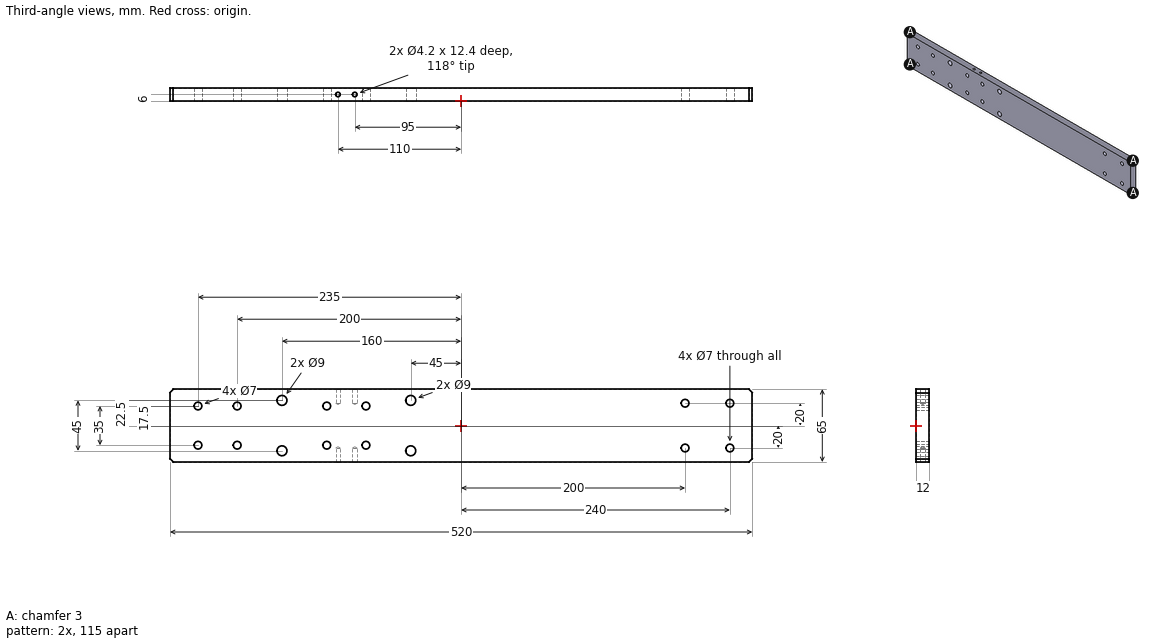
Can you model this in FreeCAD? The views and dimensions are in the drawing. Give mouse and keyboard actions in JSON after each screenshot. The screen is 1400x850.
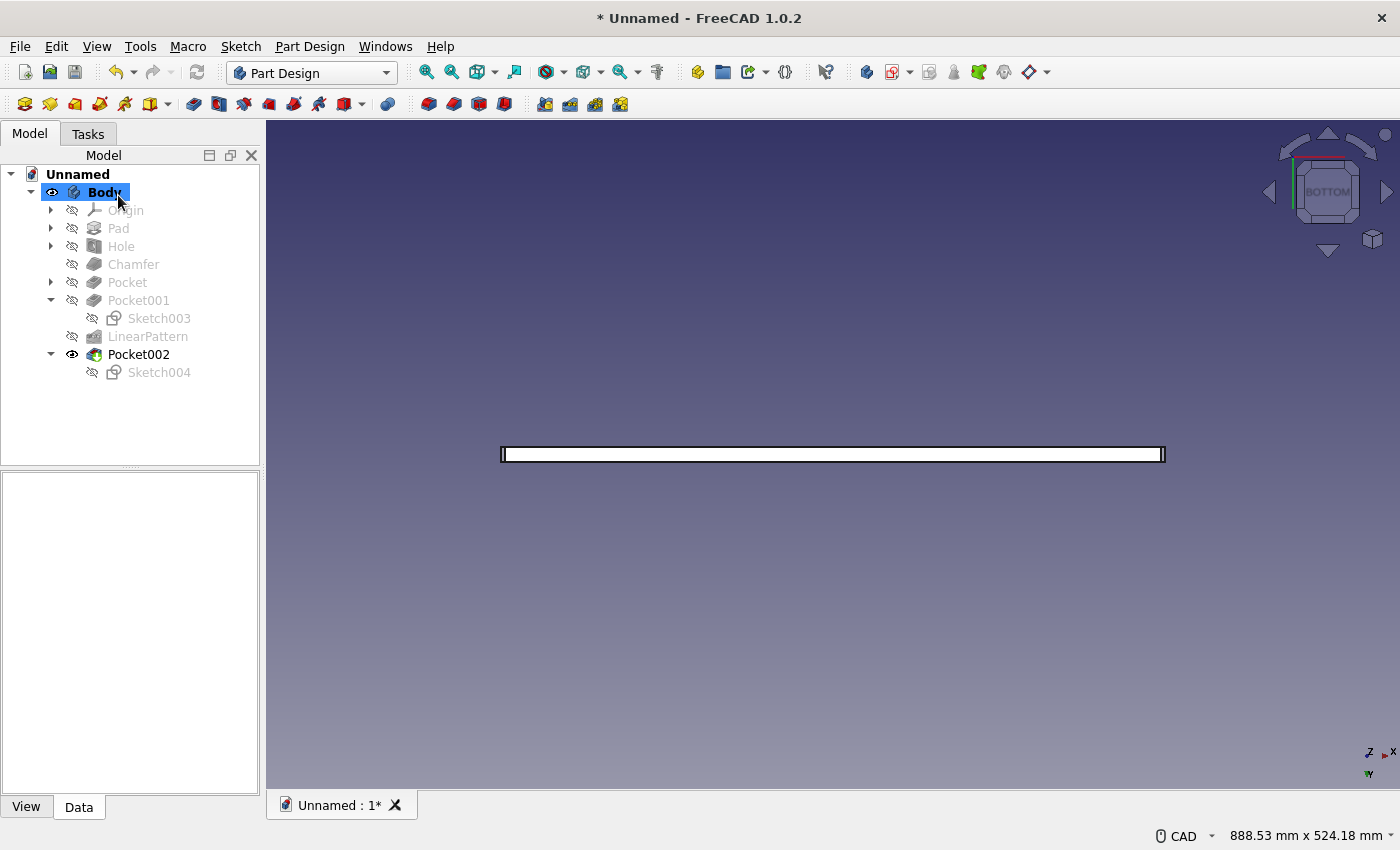
{"action": "left_click", "coordinate": [1114, 454]}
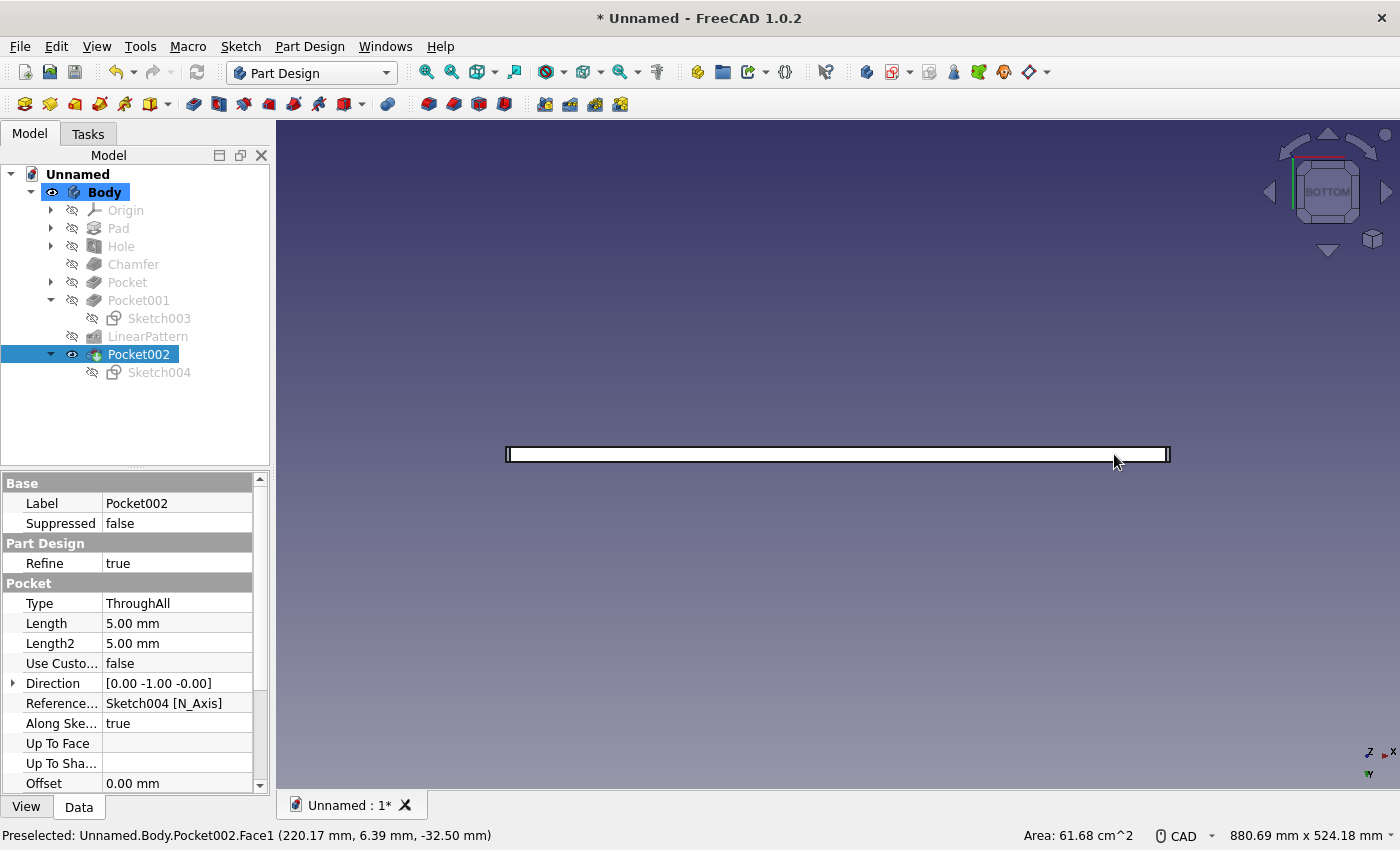
{"action": "left_click", "coordinate": [892, 72]}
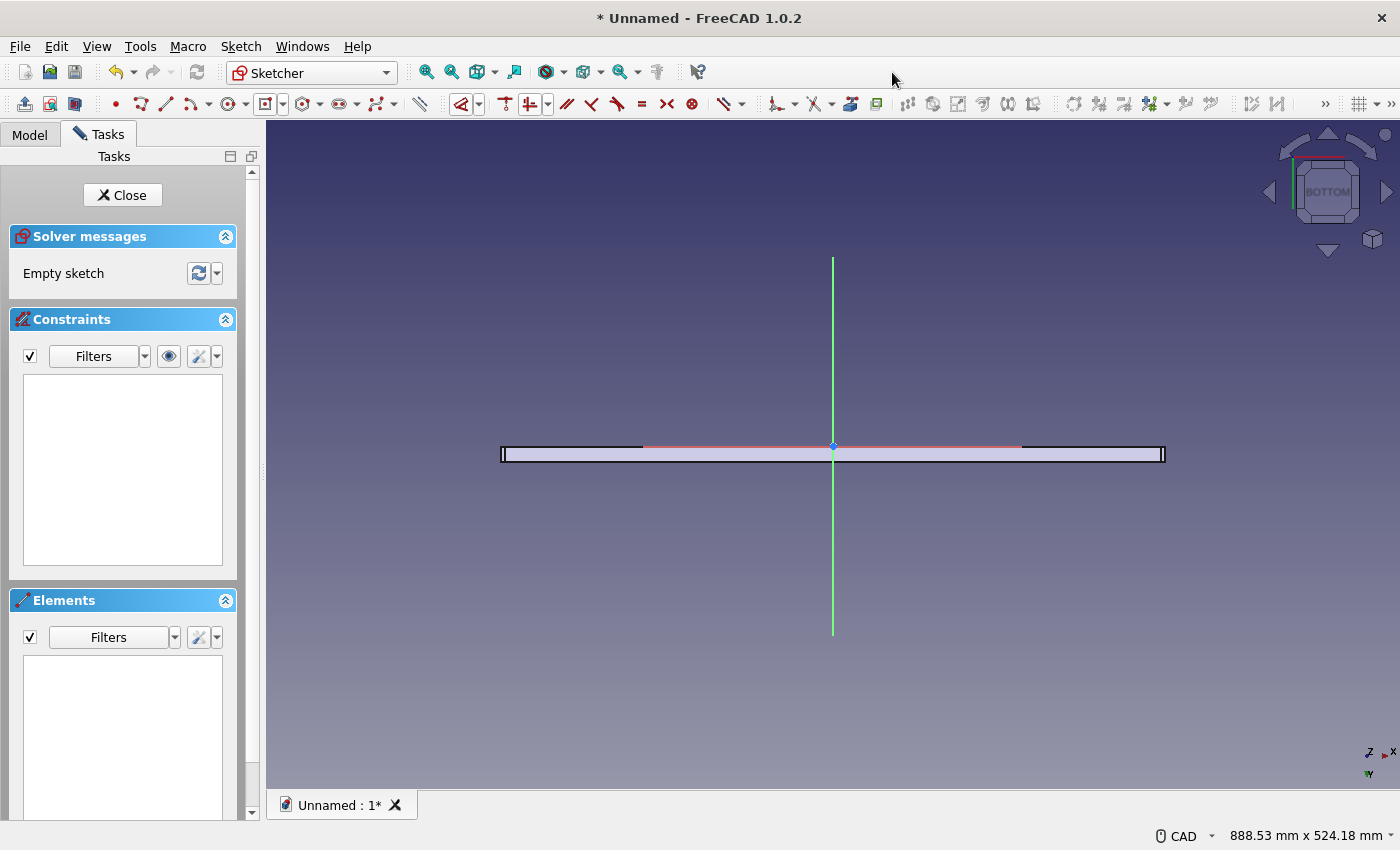
{"action": "scroll", "coordinate": [699, 455], "scroll_direction": "up", "scroll_amount": 15}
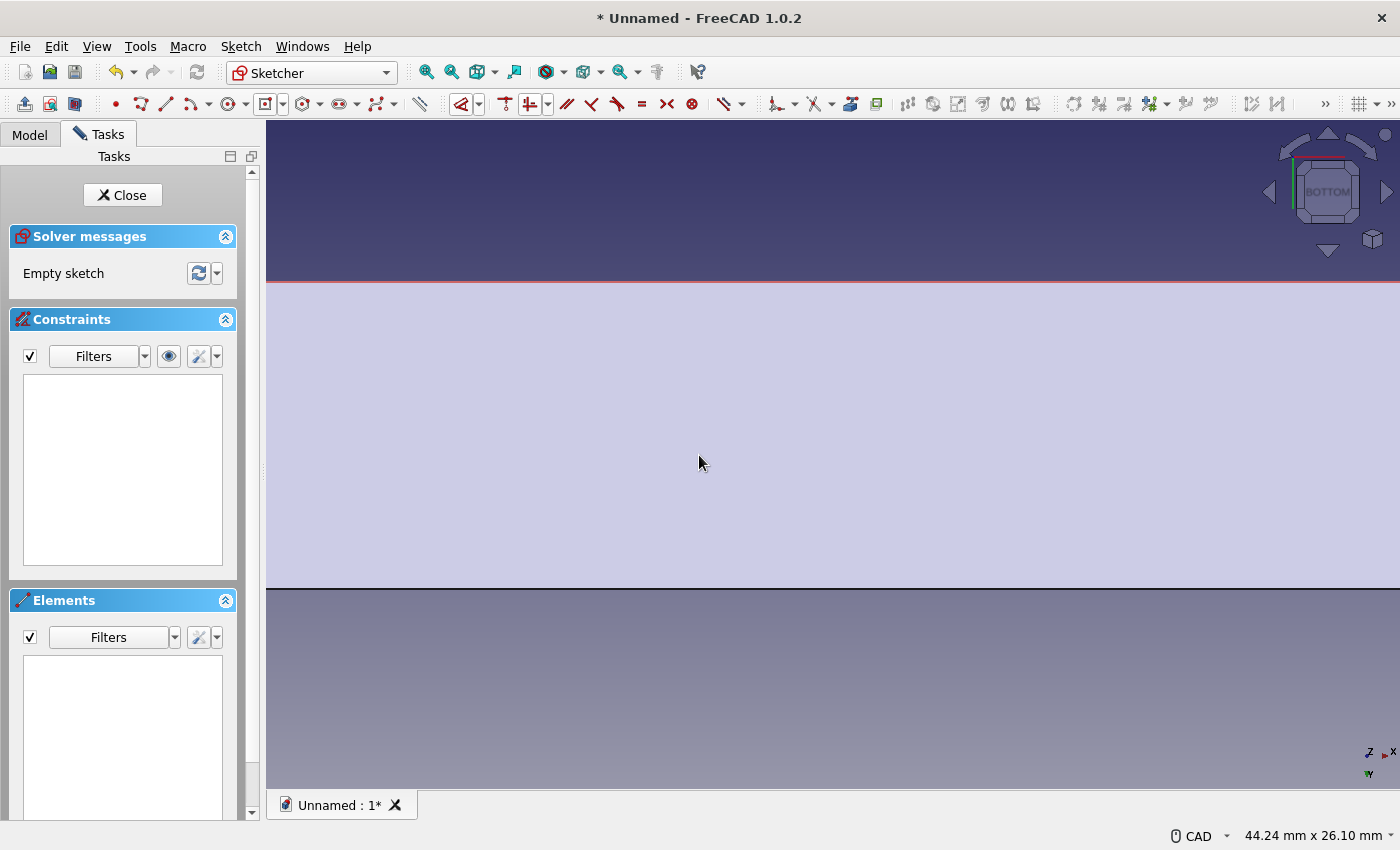
{"action": "left_click", "coordinate": [228, 104]}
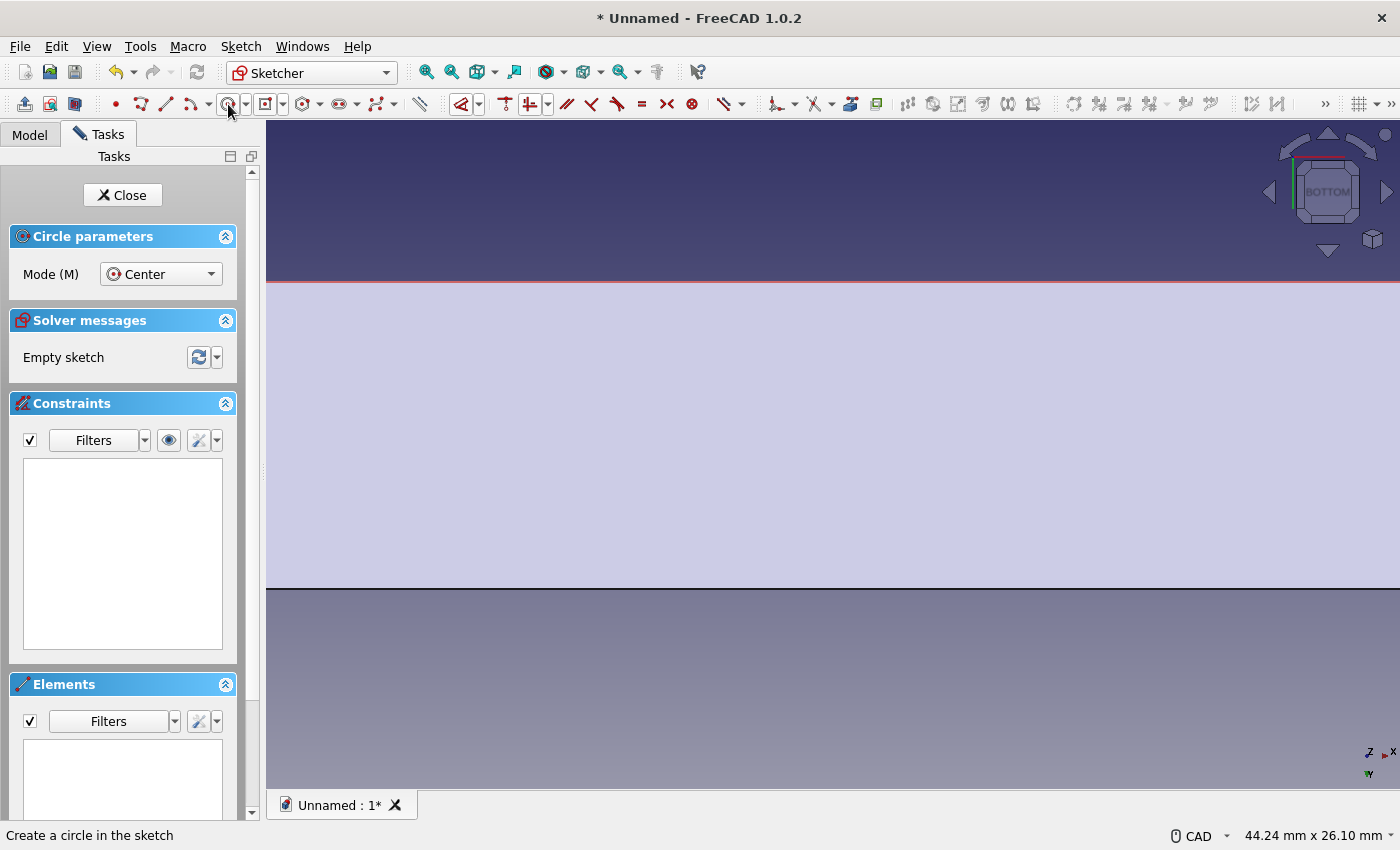
{"action": "left_click", "coordinate": [948, 435]}
{"action": "left_click", "coordinate": [986, 397]}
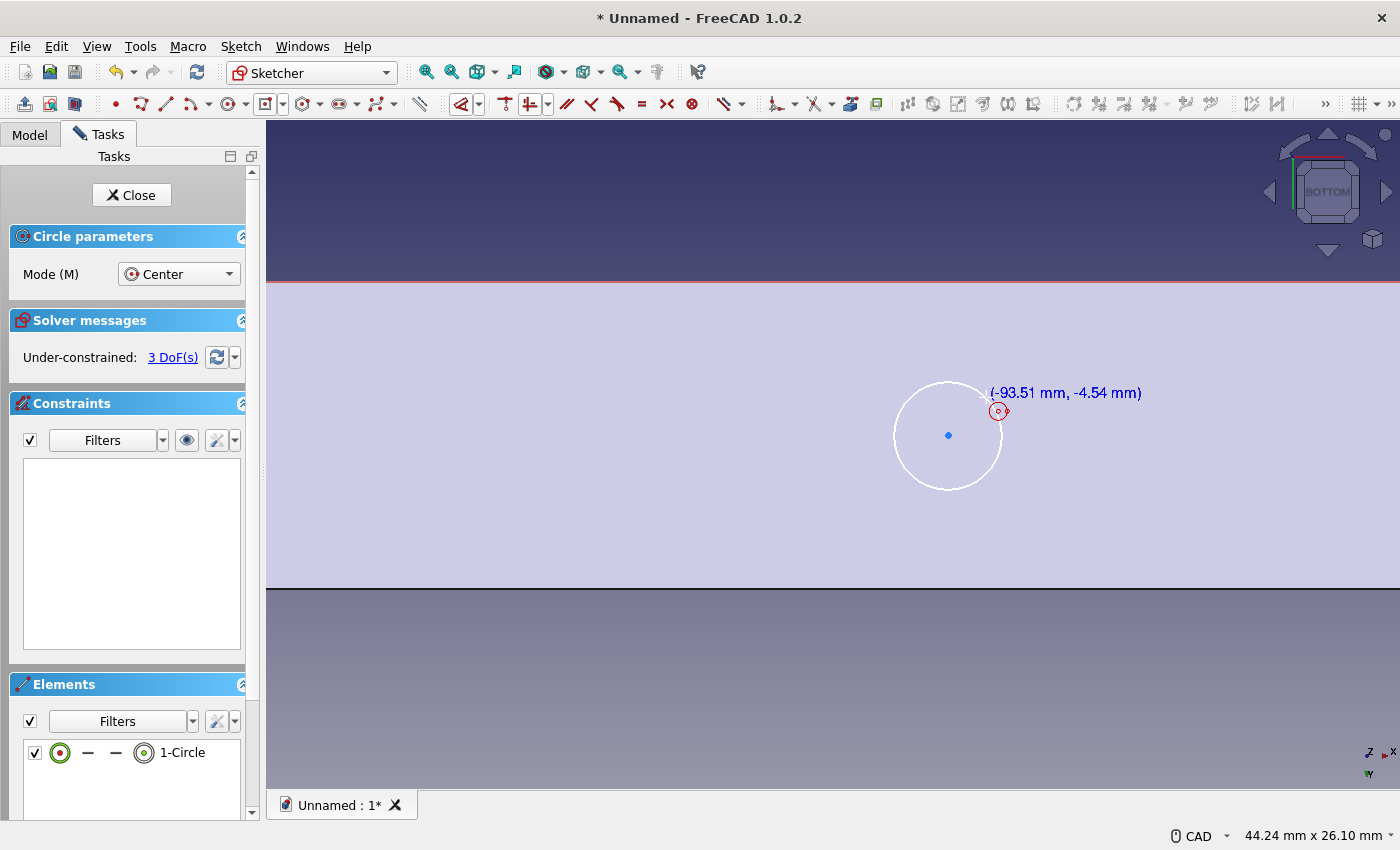
{"action": "left_click", "coordinate": [563, 435]}
{"action": "left_click", "coordinate": [601, 397]}
{"action": "key", "text": "Escape"}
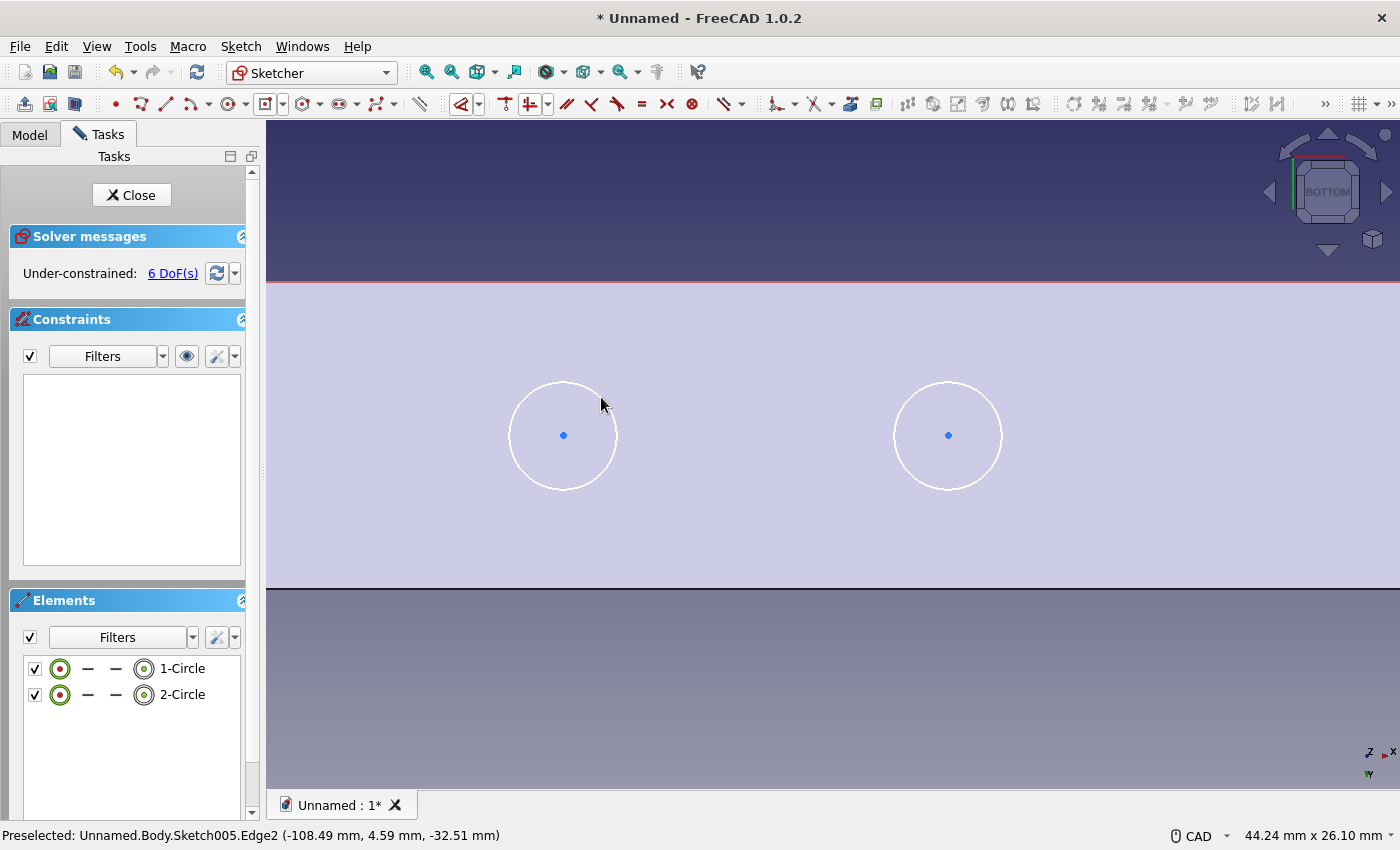
{"action": "left_click", "coordinate": [986, 398]}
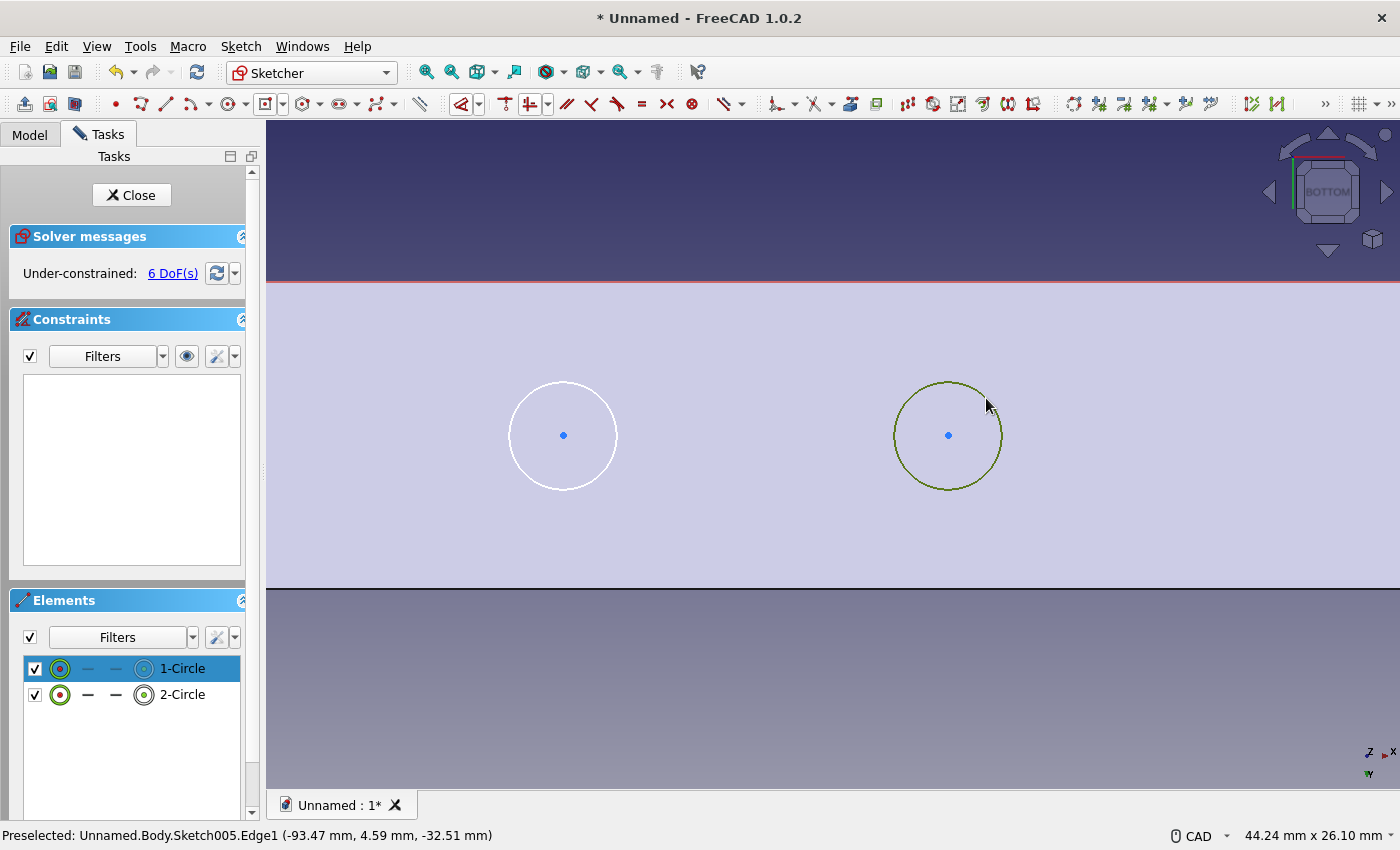
{"action": "left_click", "coordinate": [601, 398]}